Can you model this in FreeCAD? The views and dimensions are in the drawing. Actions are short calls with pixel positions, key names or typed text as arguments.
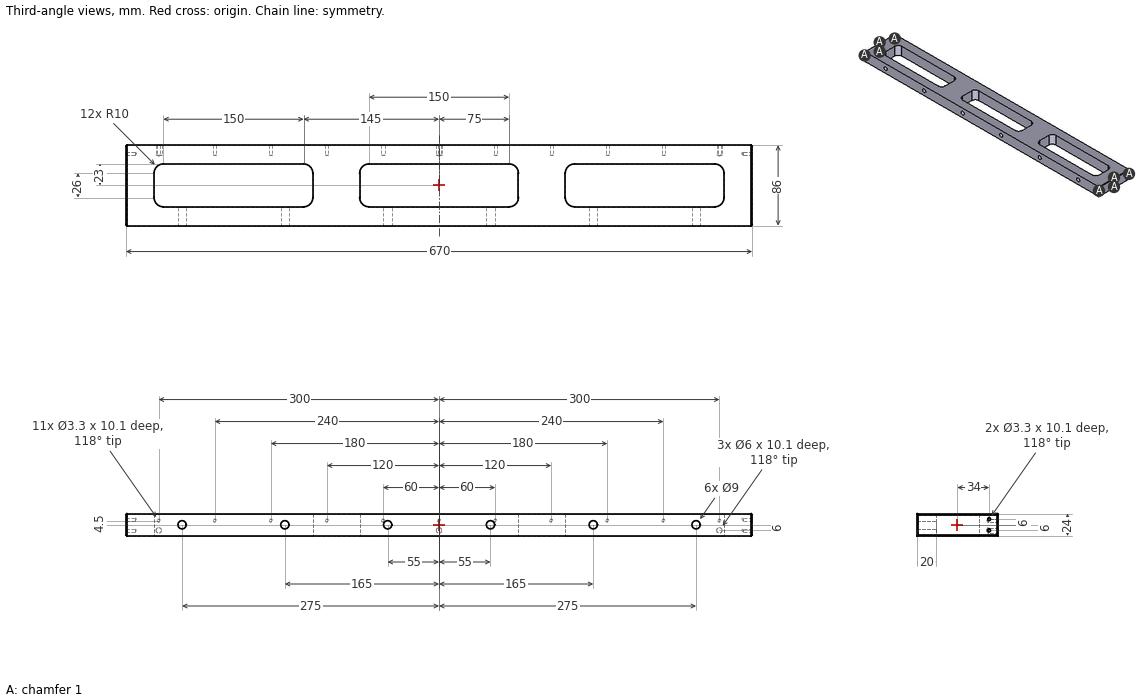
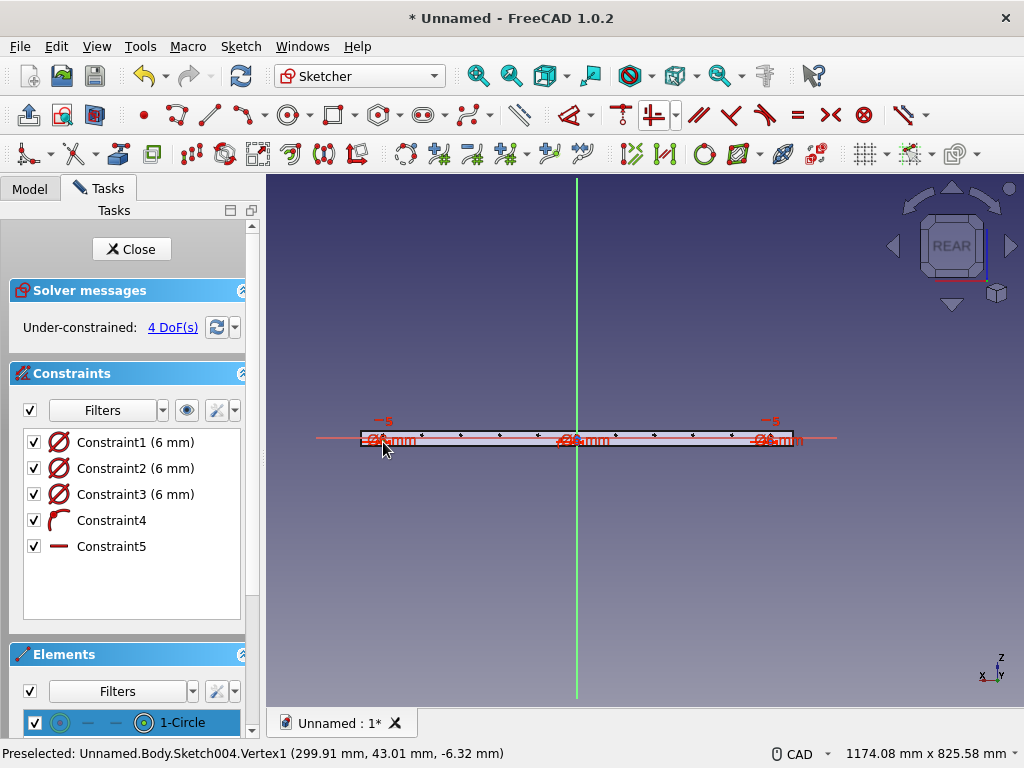
scroll(577, 442, up, 6)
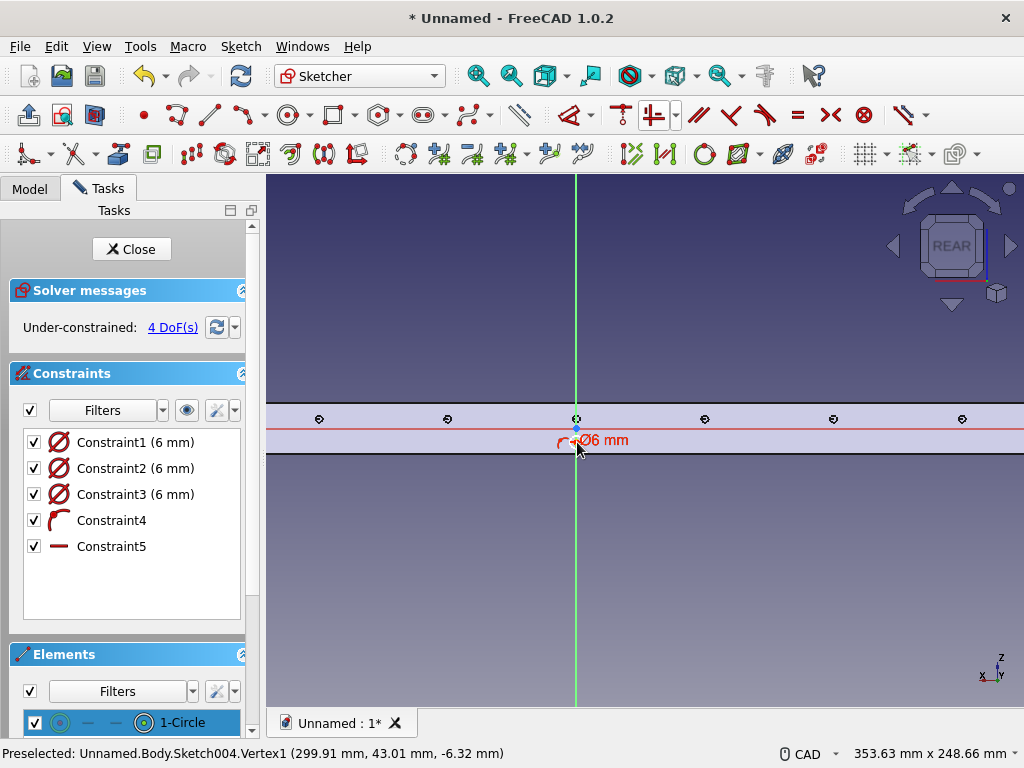
click(576, 442)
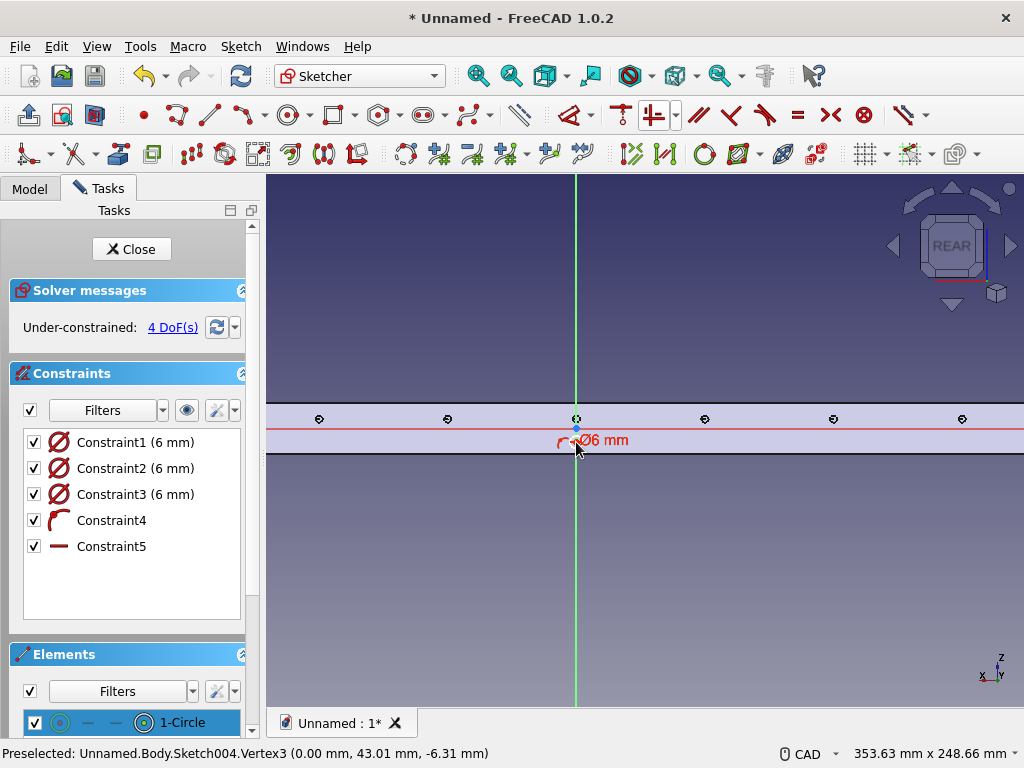
key(h)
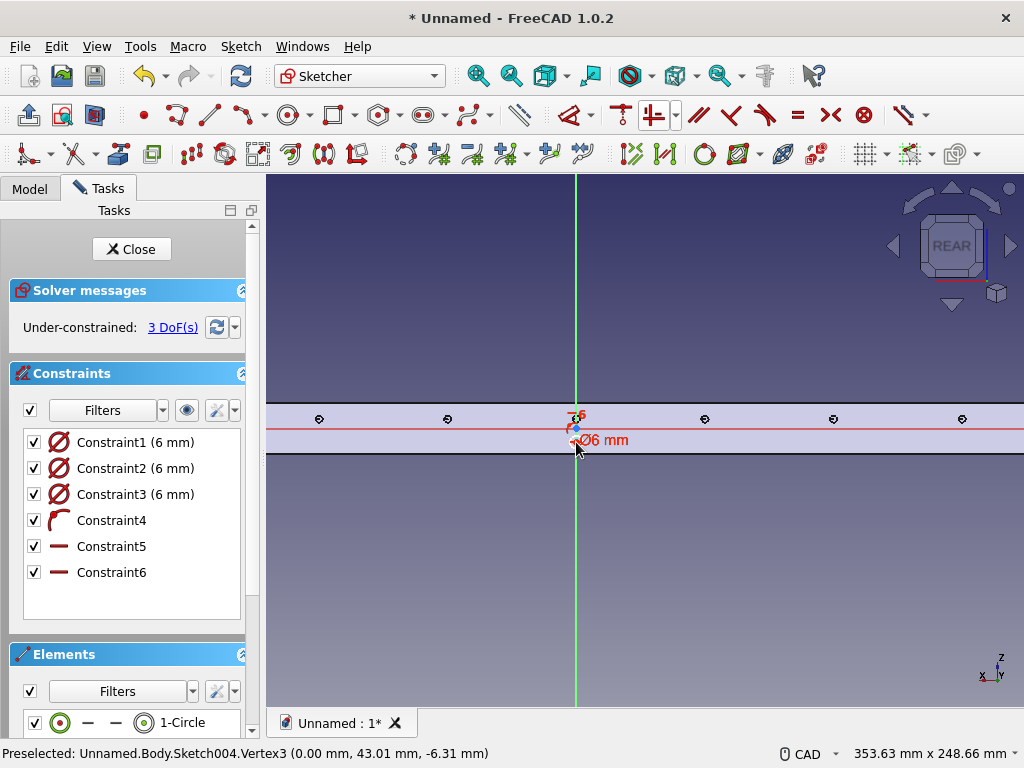
key(d)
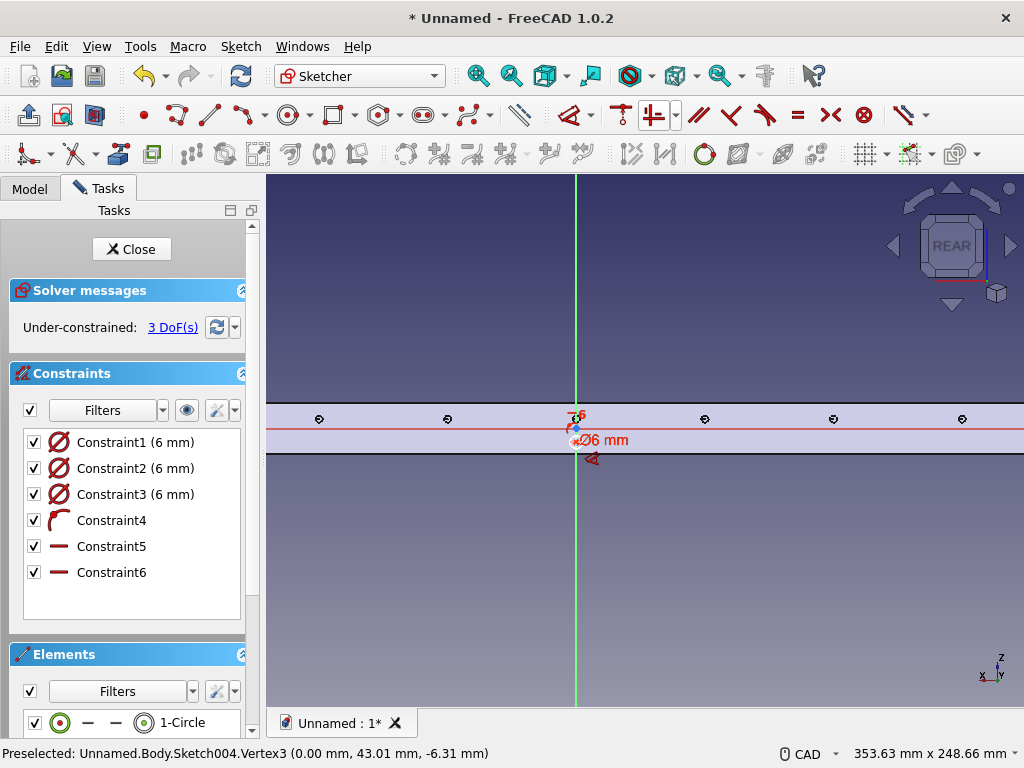
scroll(577, 441, down, 6)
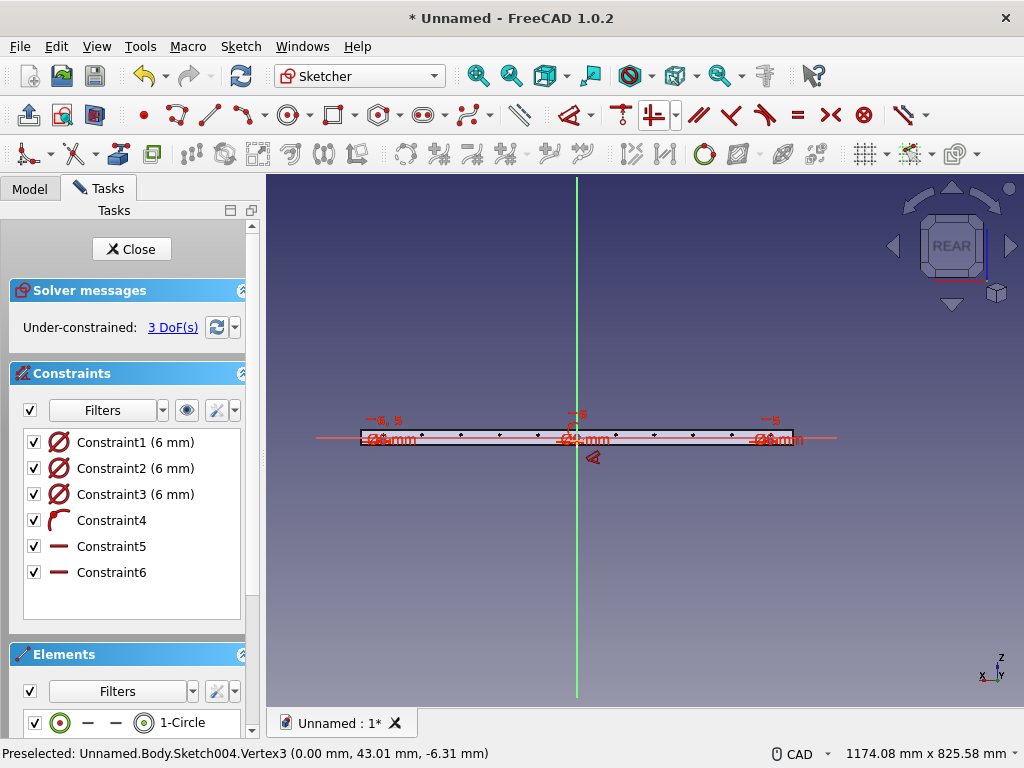
scroll(383, 442, up, 12)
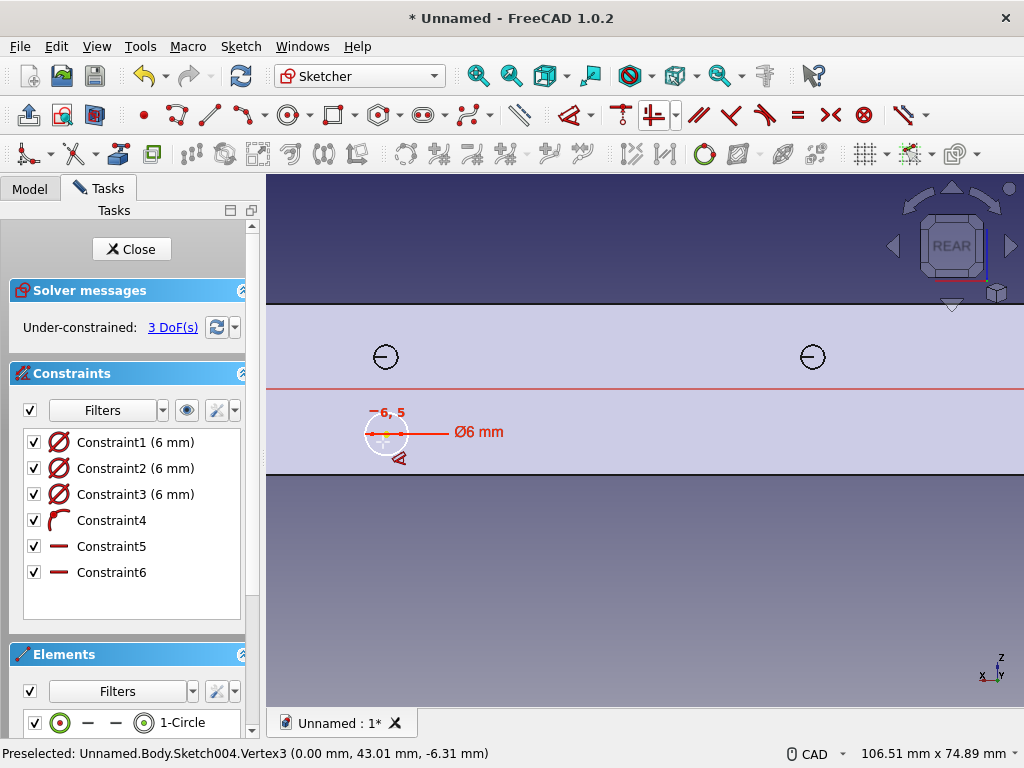
click(387, 434)
click(353, 412)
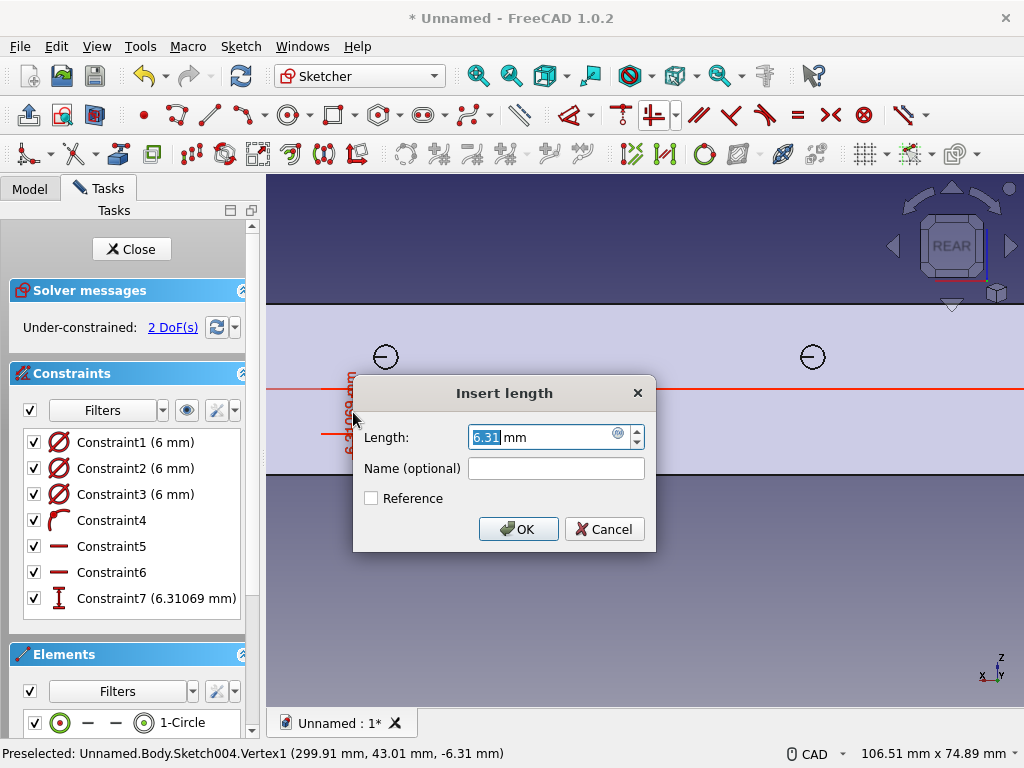
text(6)
key(Return)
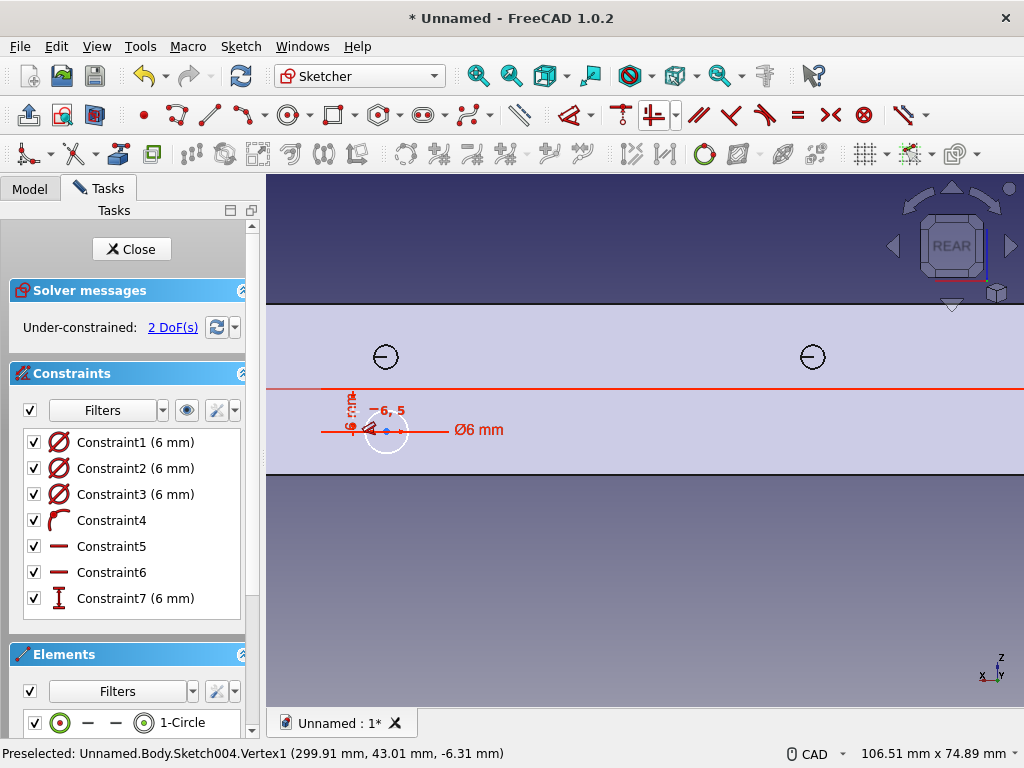
scroll(383, 442, down, 12)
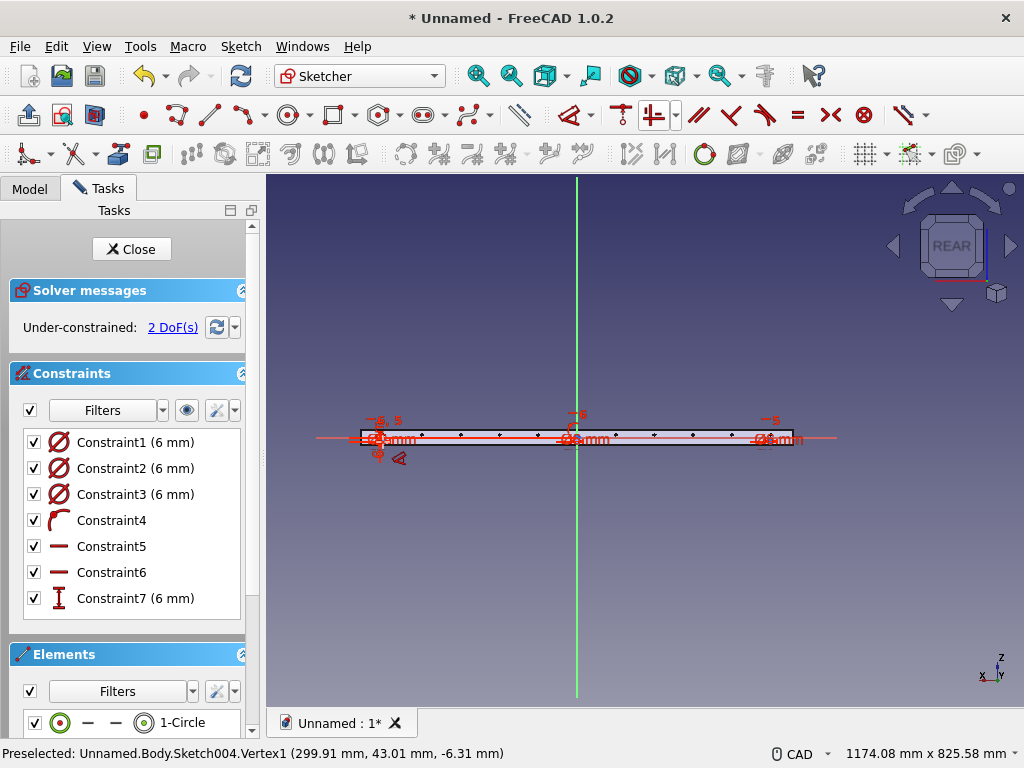
click(383, 442)
click(480, 404)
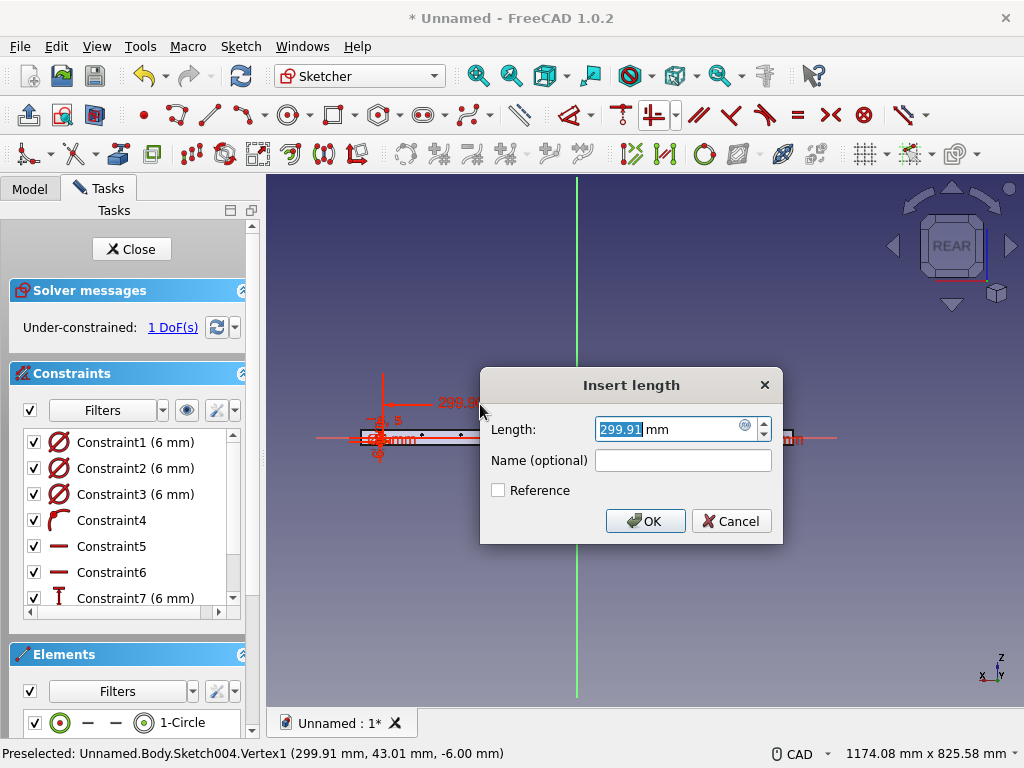
text(300)
key(Return)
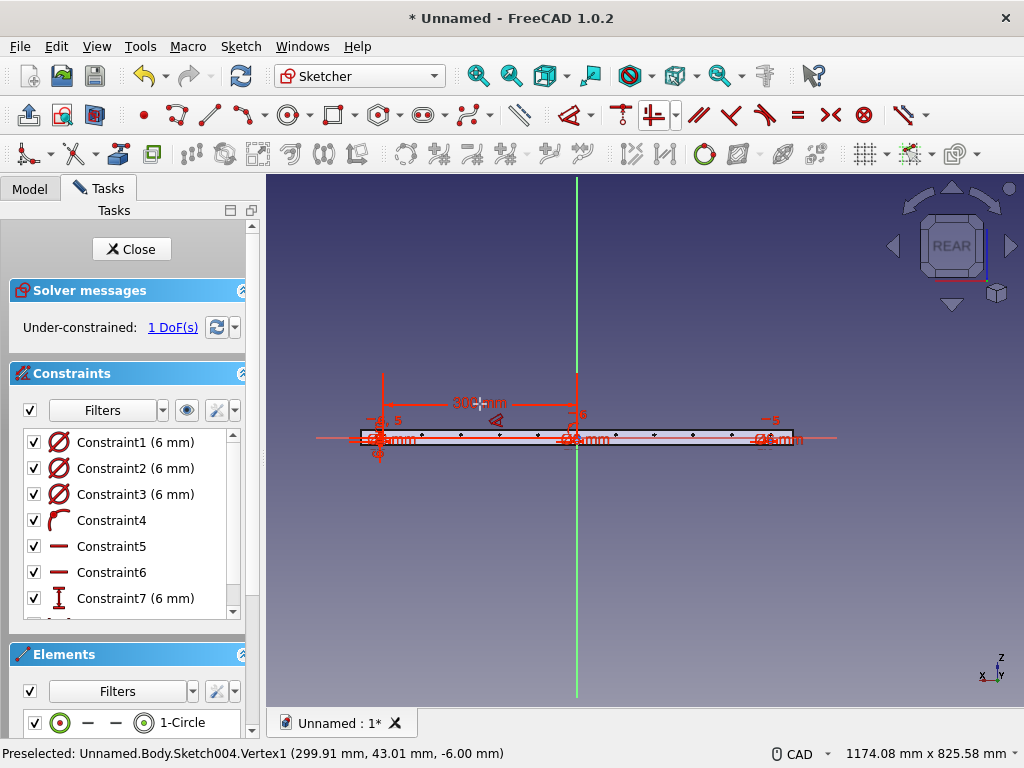
click(771, 442)
click(674, 404)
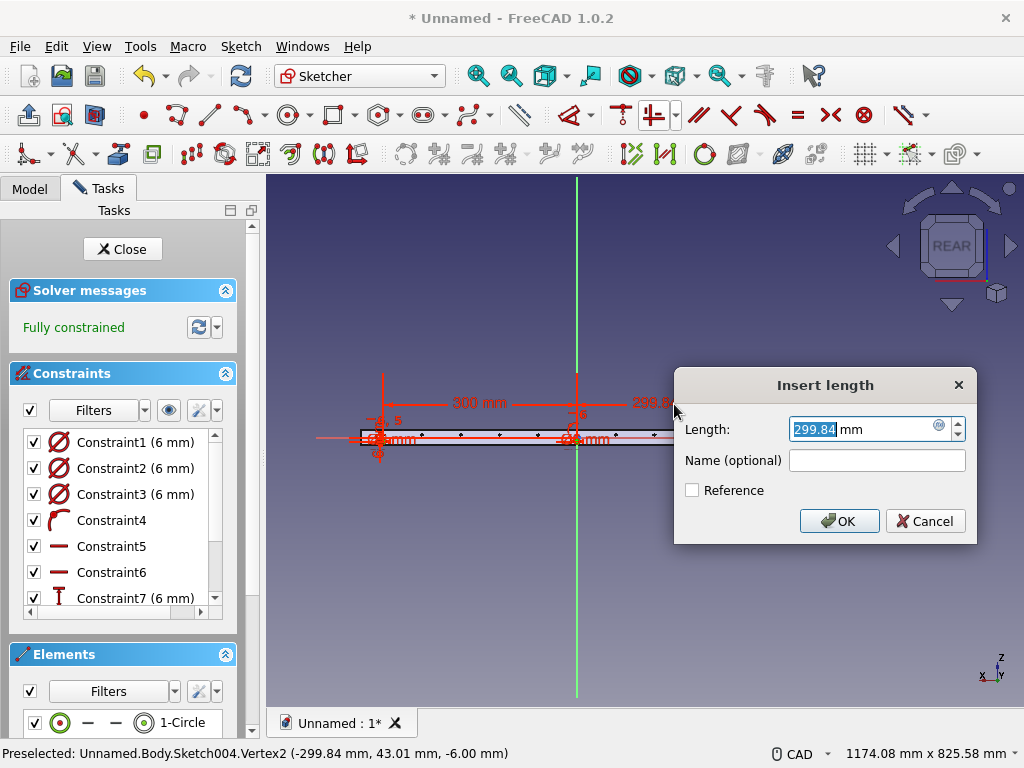
text(300)
key(Return)
key(Escape)